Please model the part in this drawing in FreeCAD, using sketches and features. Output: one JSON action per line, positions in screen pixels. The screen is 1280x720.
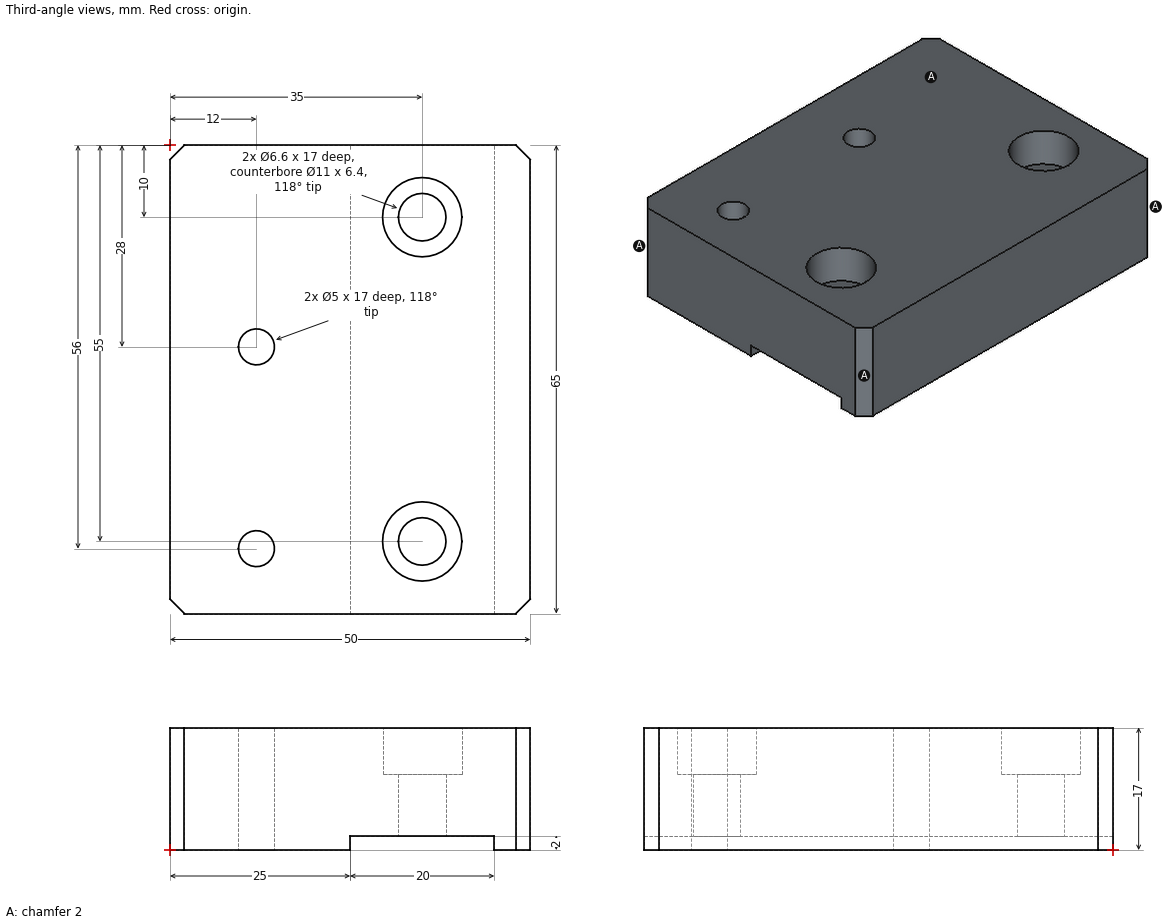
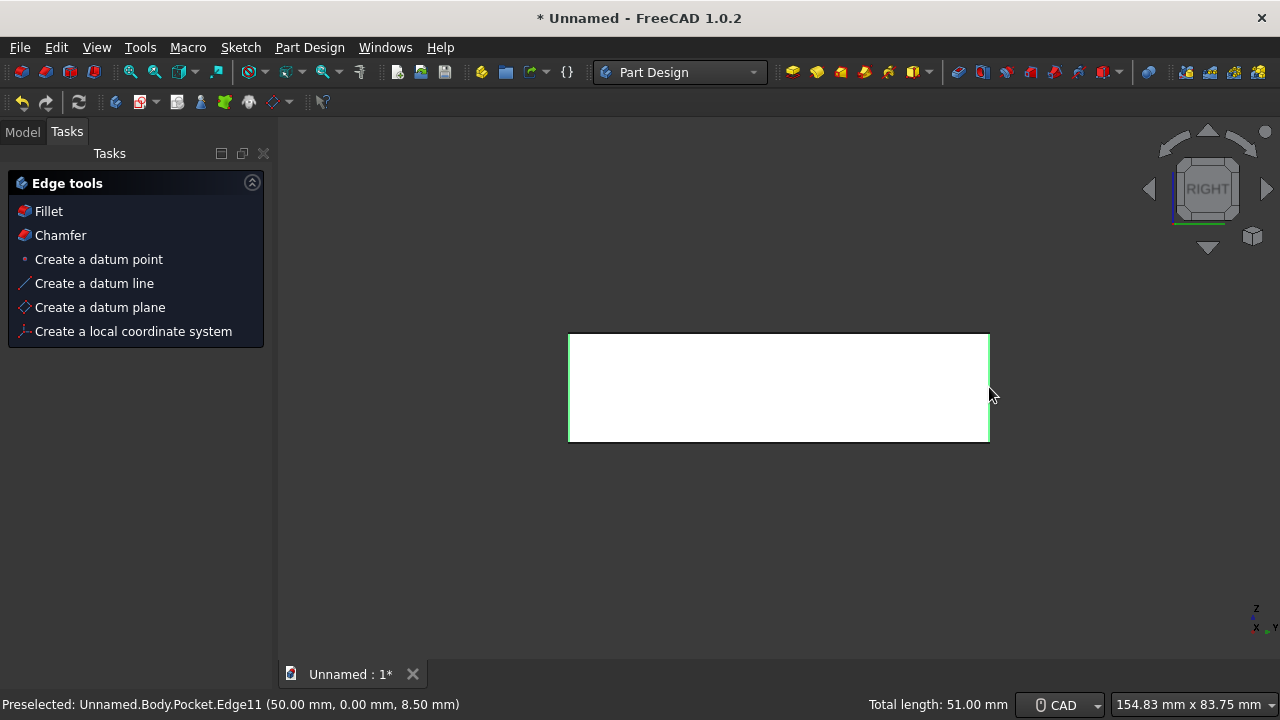
{"action": "key", "text": "5"}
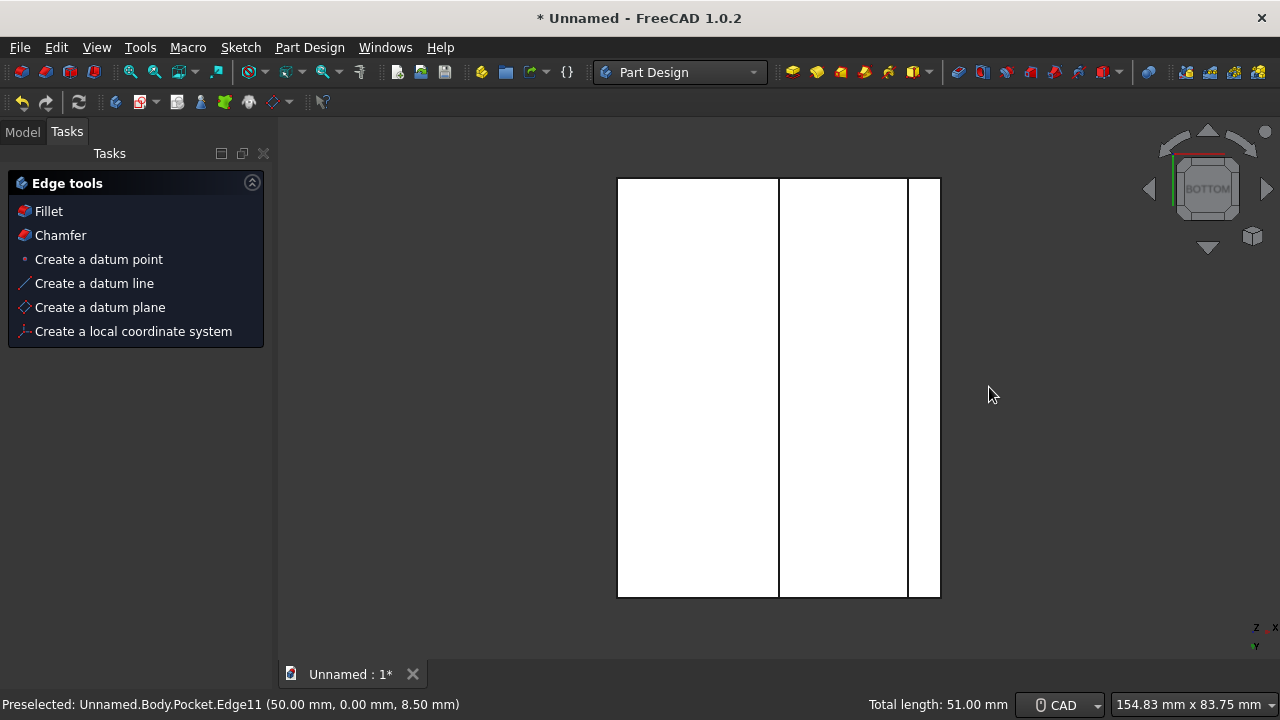
{"action": "key", "text": "4"}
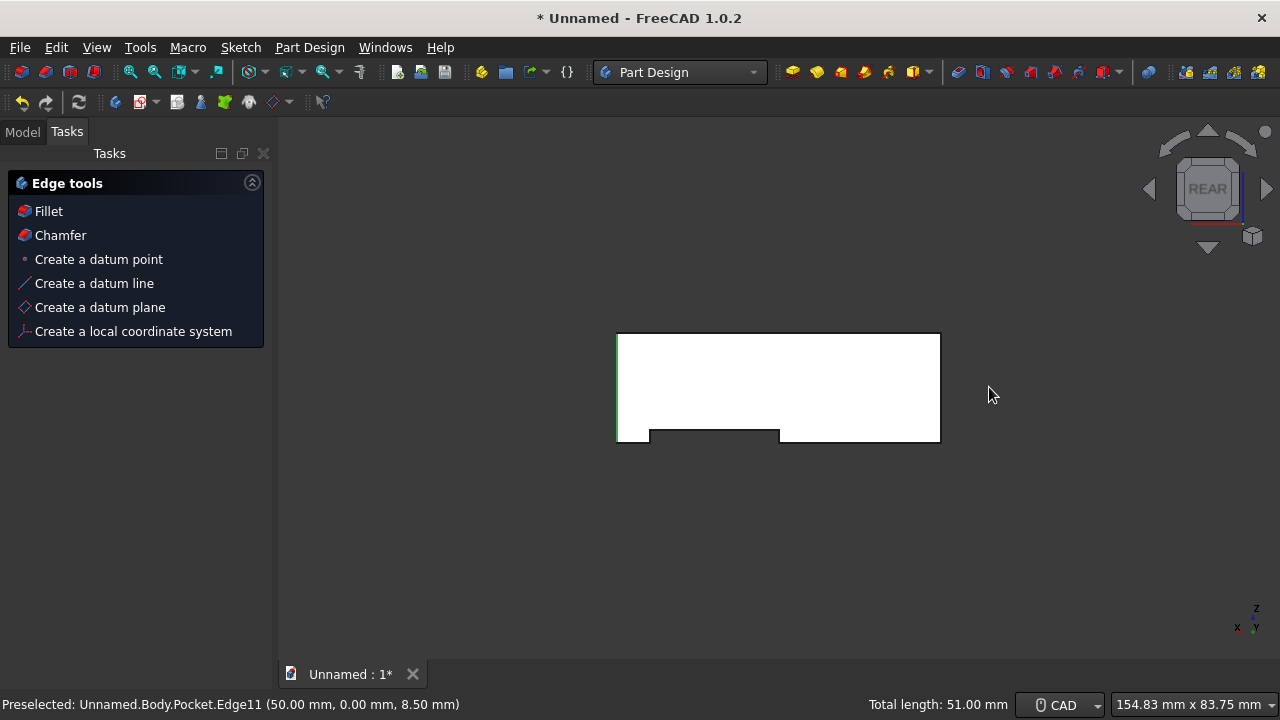
{"action": "left_click", "coordinate": [132, 72]}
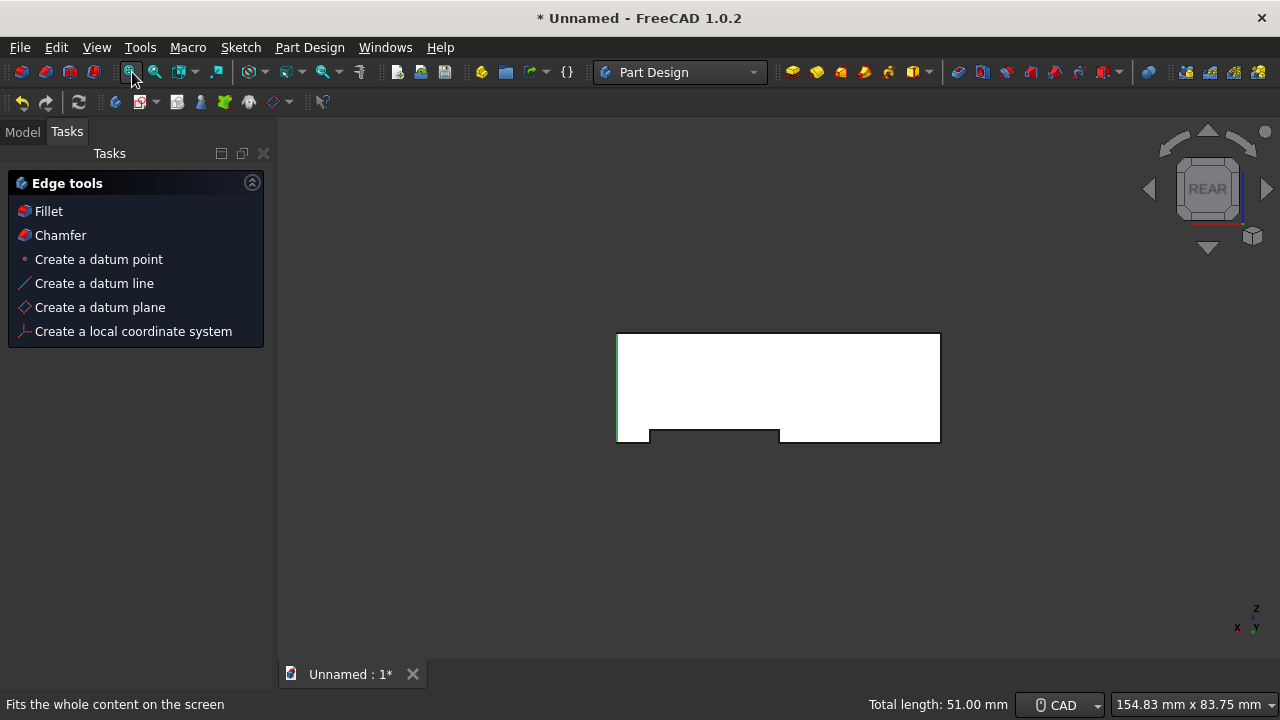
{"action": "left_click", "coordinate": [941, 387], "text": "ctrl"}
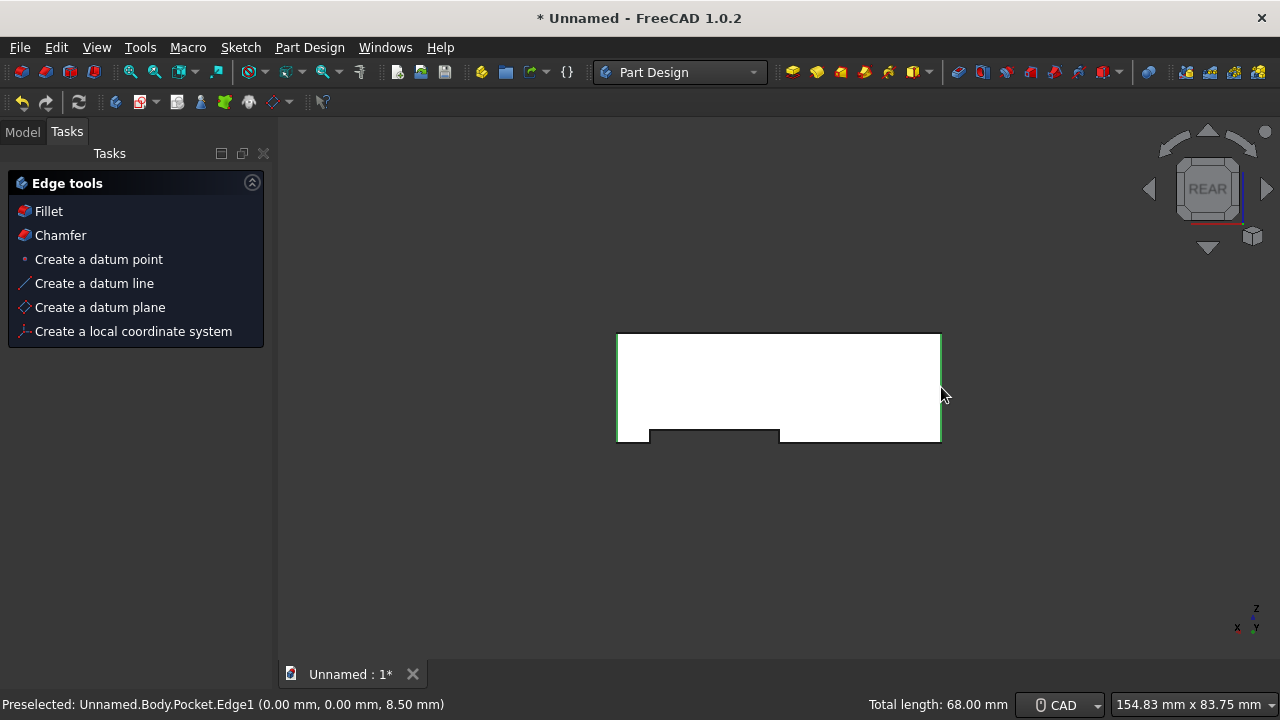
{"action": "left_click", "coordinate": [46, 72]}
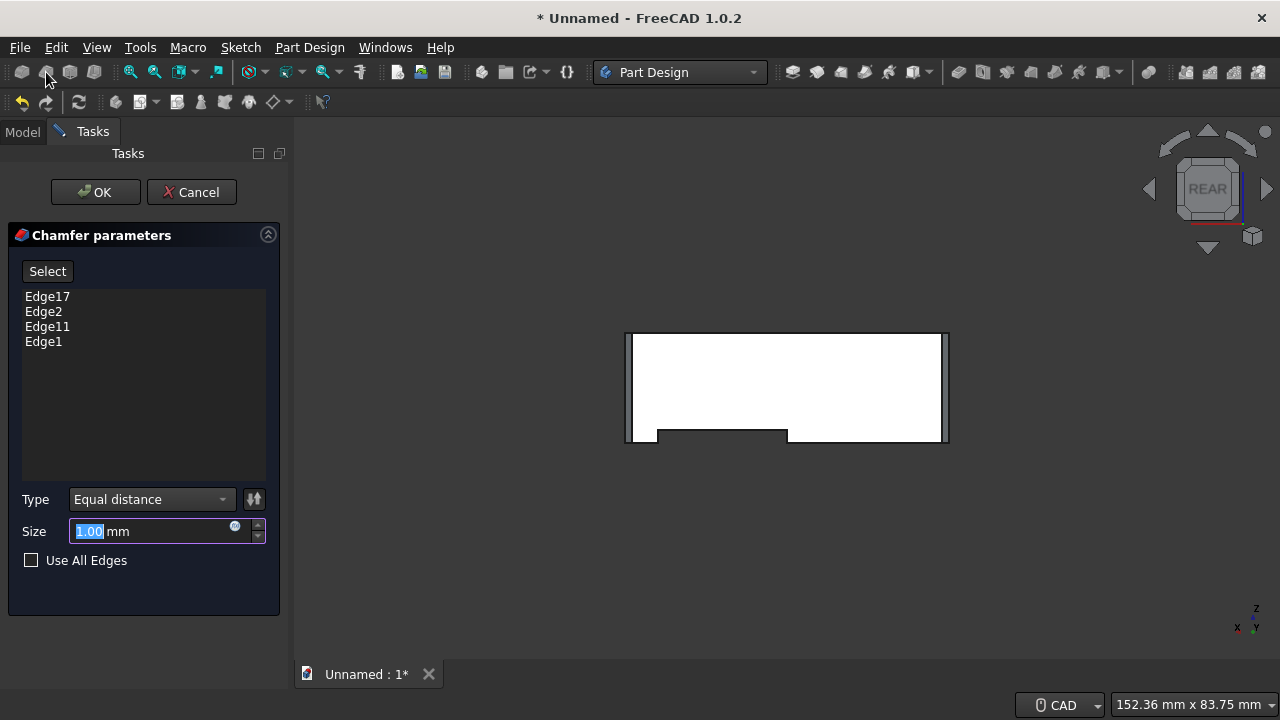
{"action": "type", "text": "2"}
{"action": "key", "text": "Tab"}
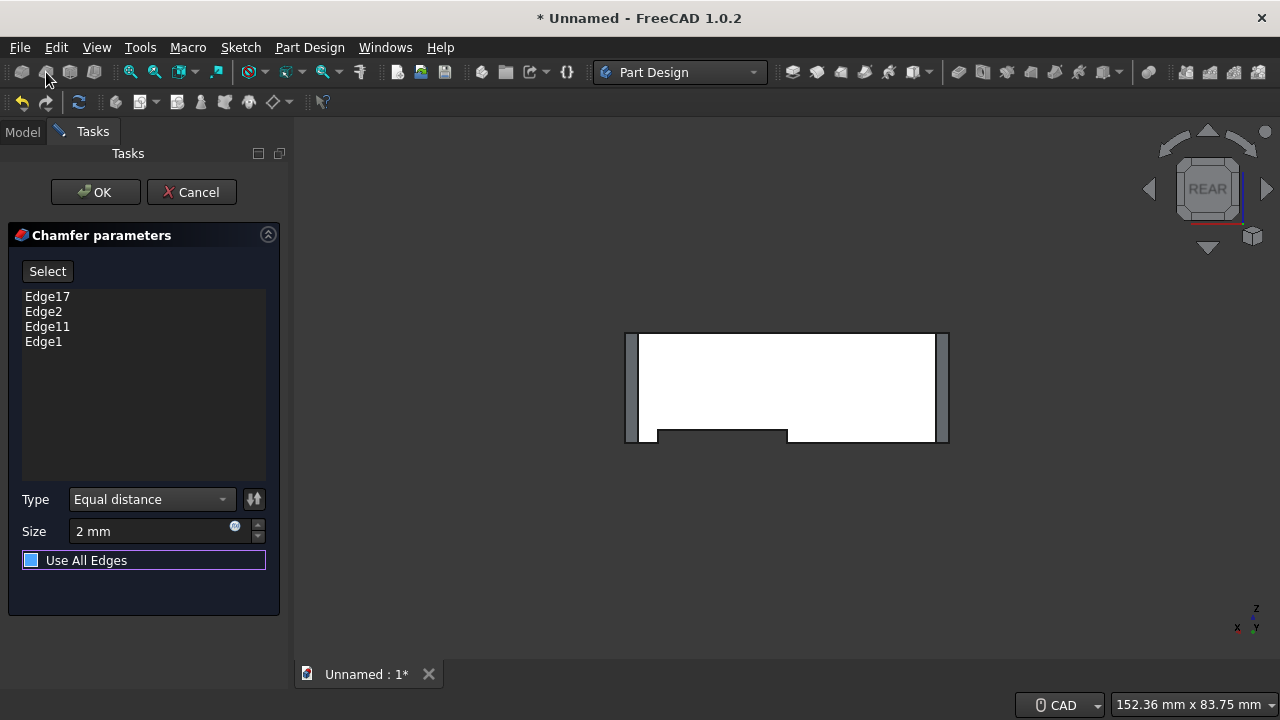
{"action": "left_click", "coordinate": [96, 192]}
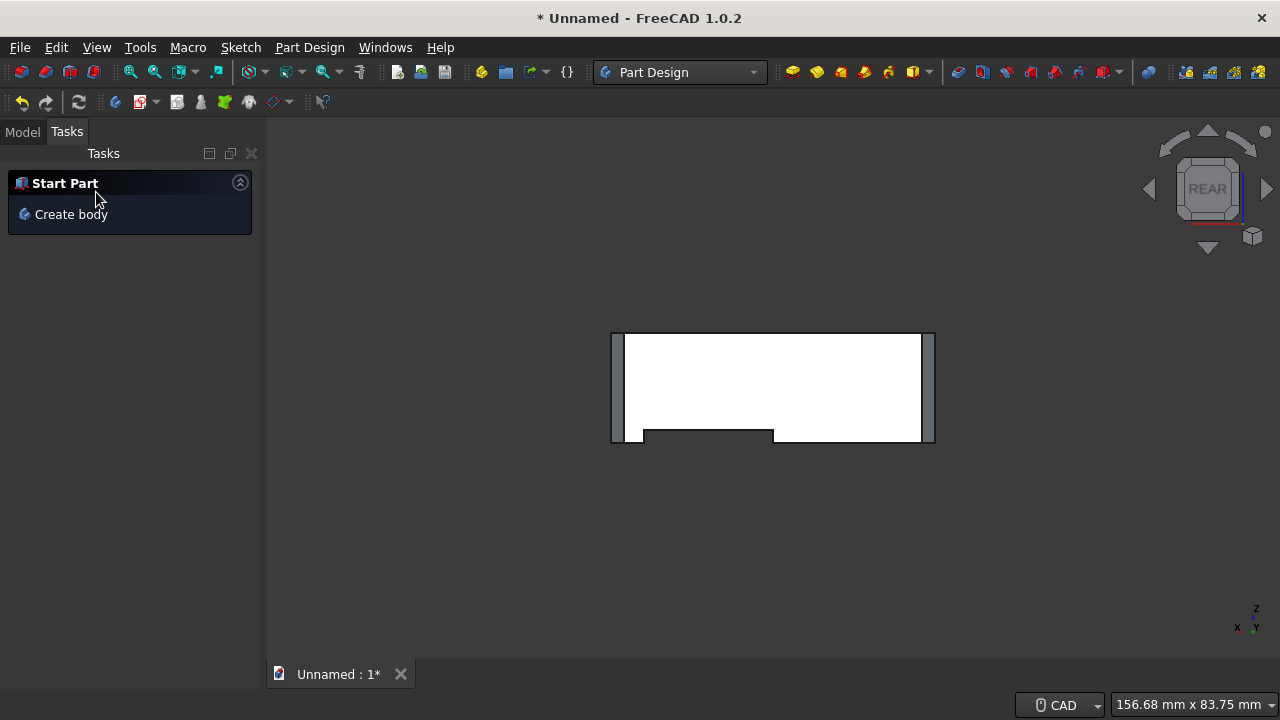
{"action": "left_click", "coordinate": [132, 72]}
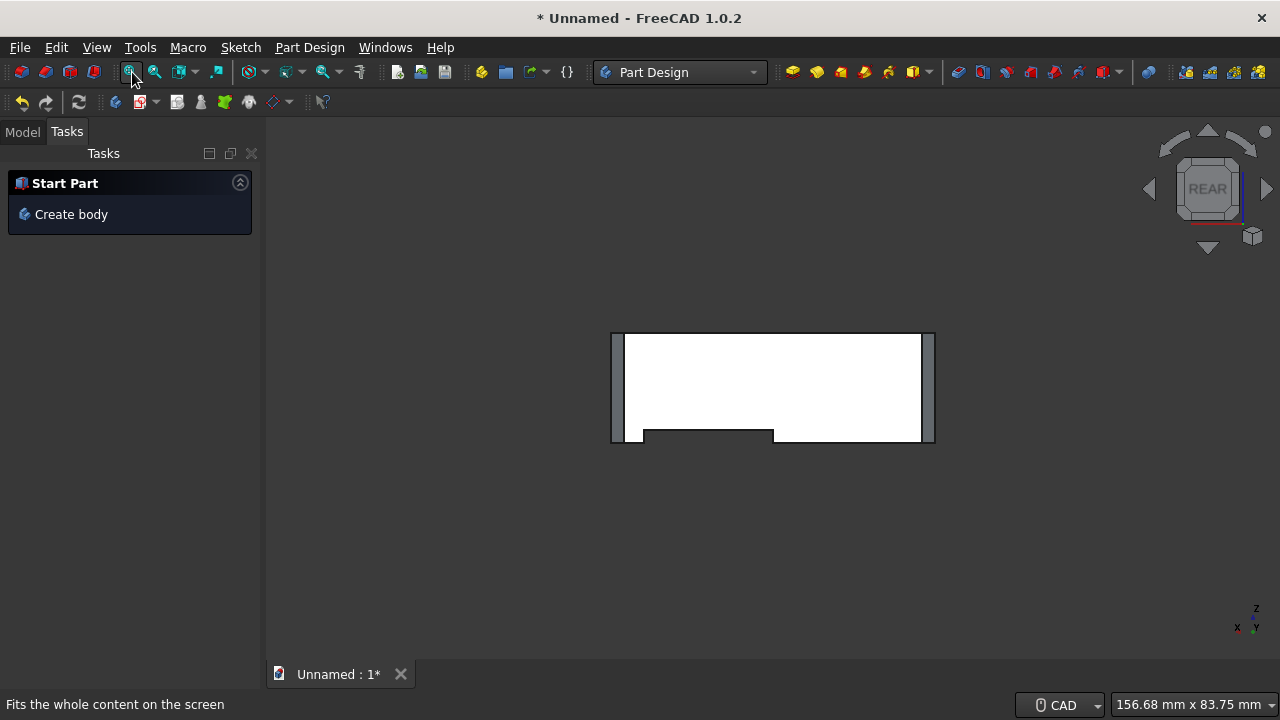
{"action": "key", "text": "0"}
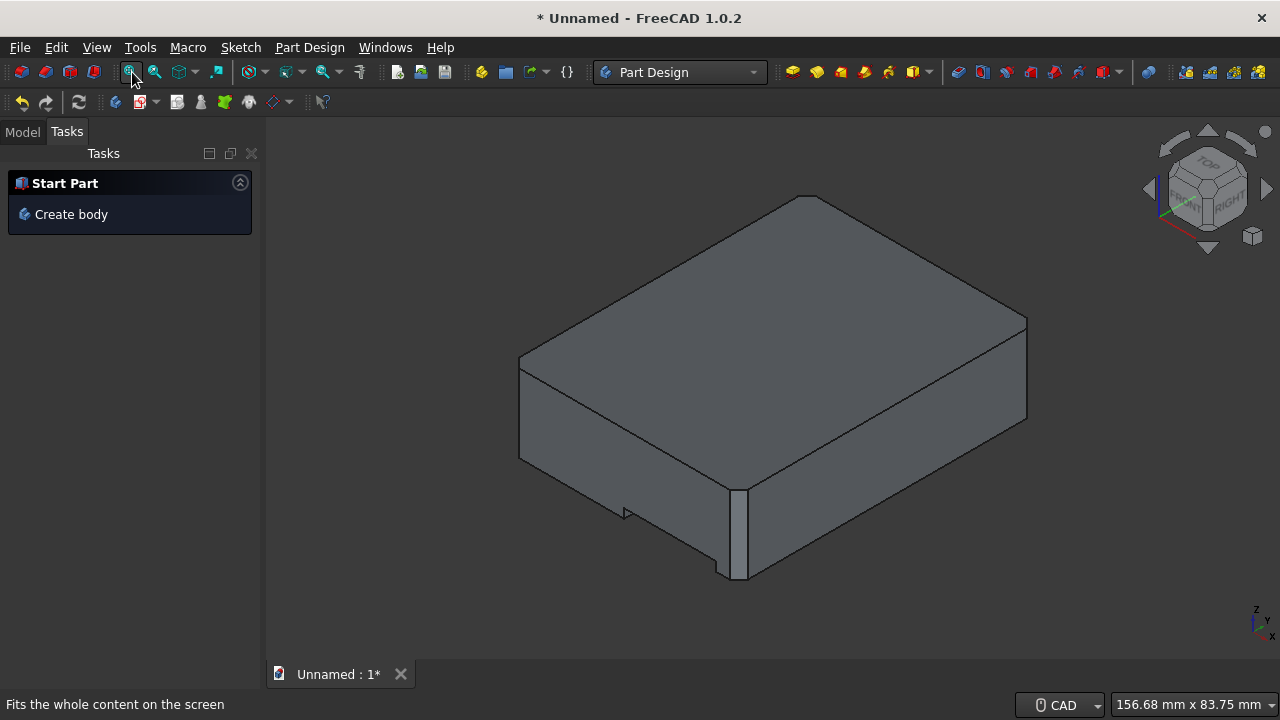
{"action": "left_click", "coordinate": [773, 342]}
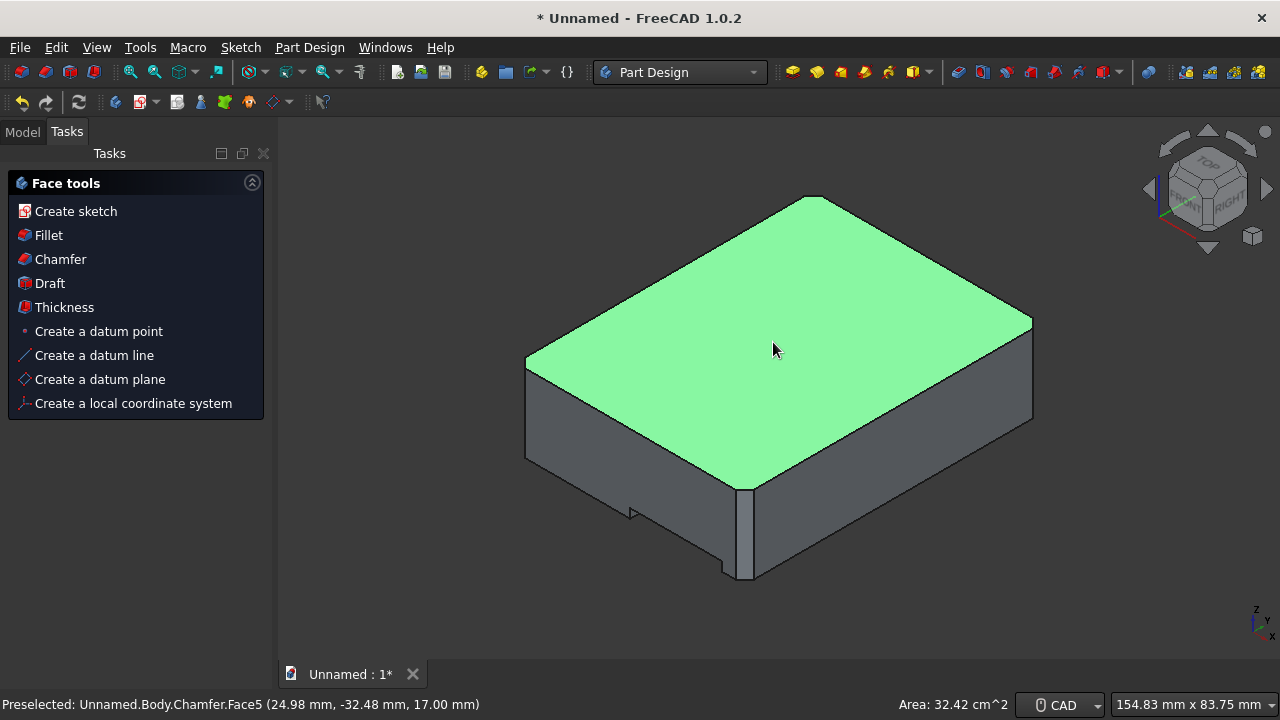
{"action": "left_click", "coordinate": [140, 102]}